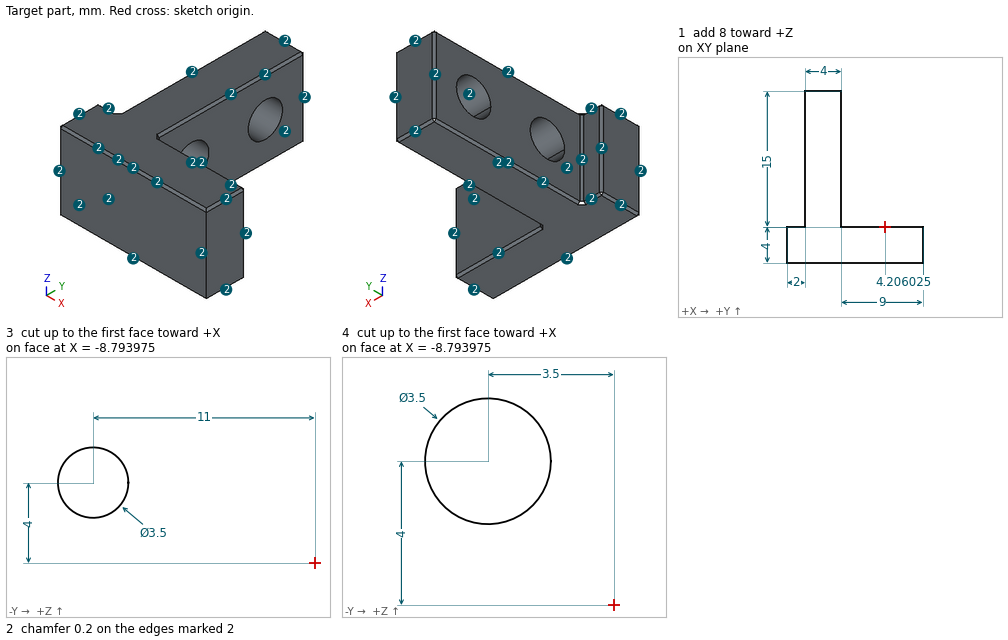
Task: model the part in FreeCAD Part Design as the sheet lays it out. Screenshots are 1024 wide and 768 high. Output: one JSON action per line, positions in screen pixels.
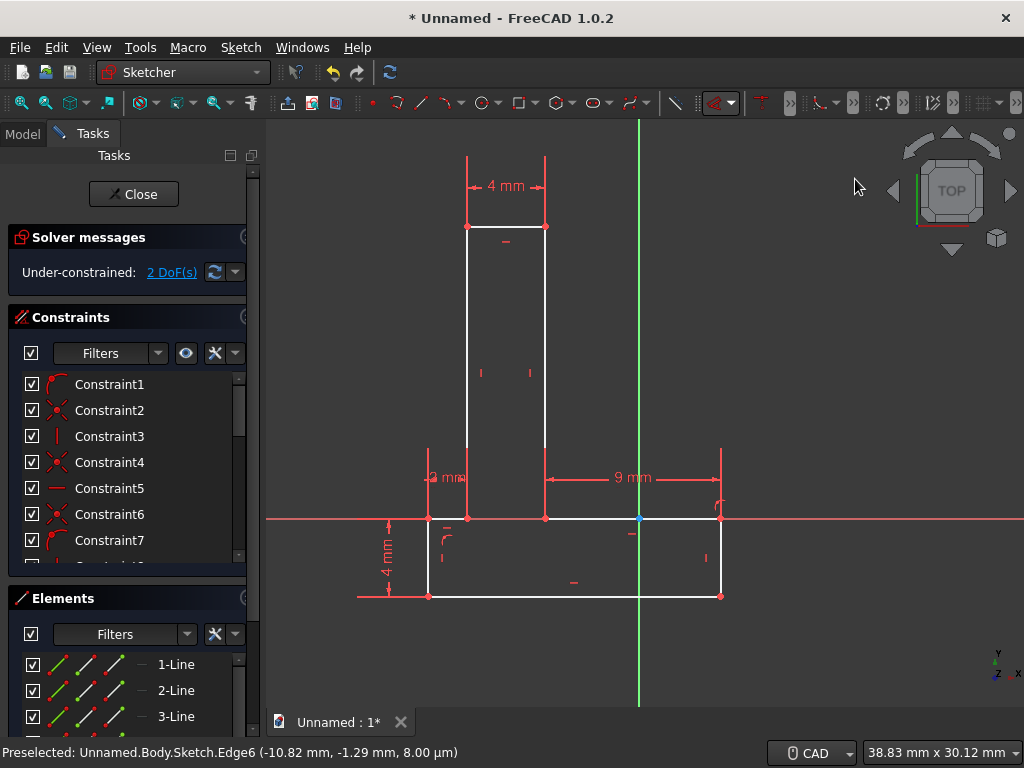
{"action": "left_click", "coordinate": [545, 431]}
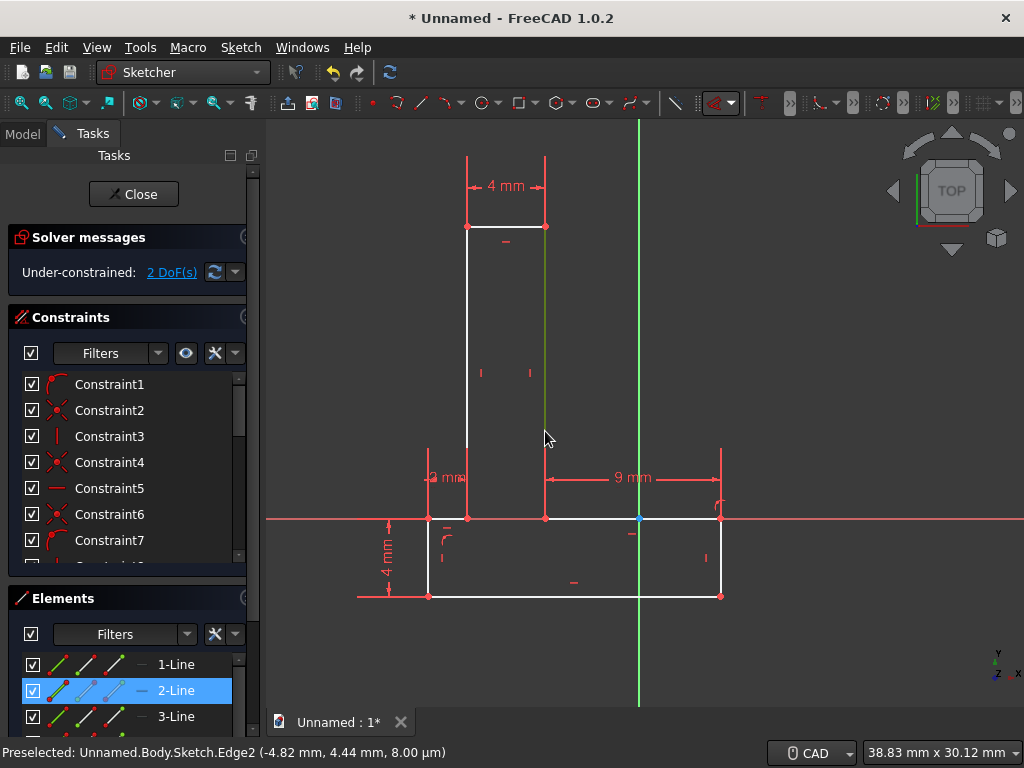
{"action": "left_click", "coordinate": [734, 104]}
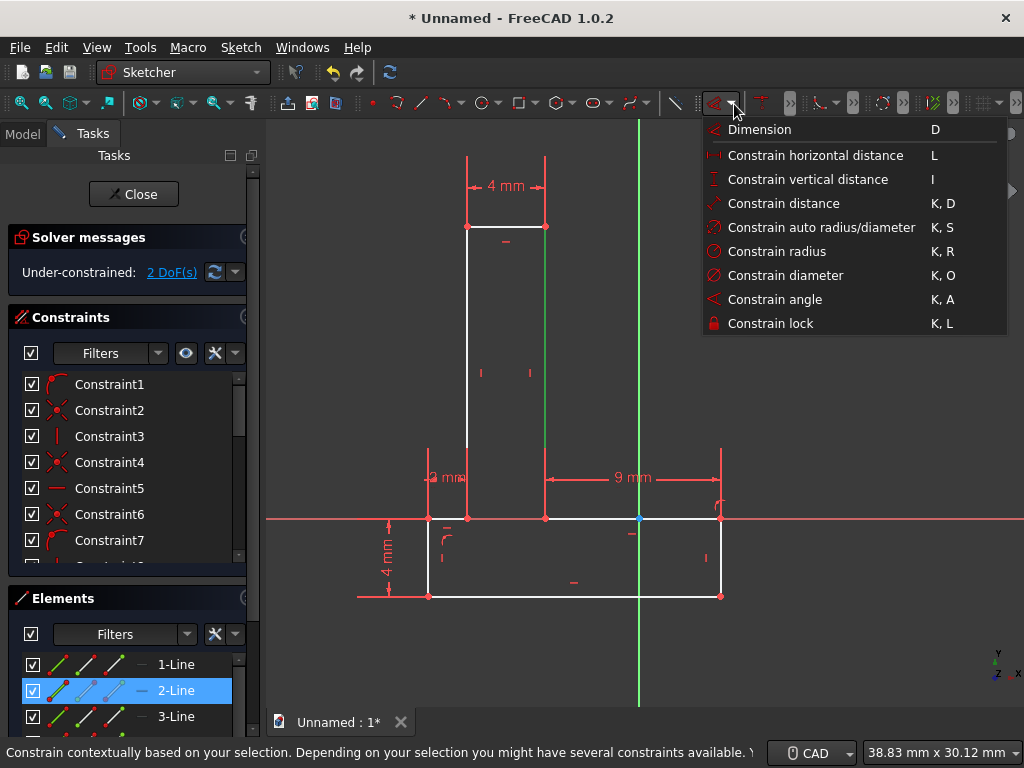
{"action": "left_click", "coordinate": [855, 179]}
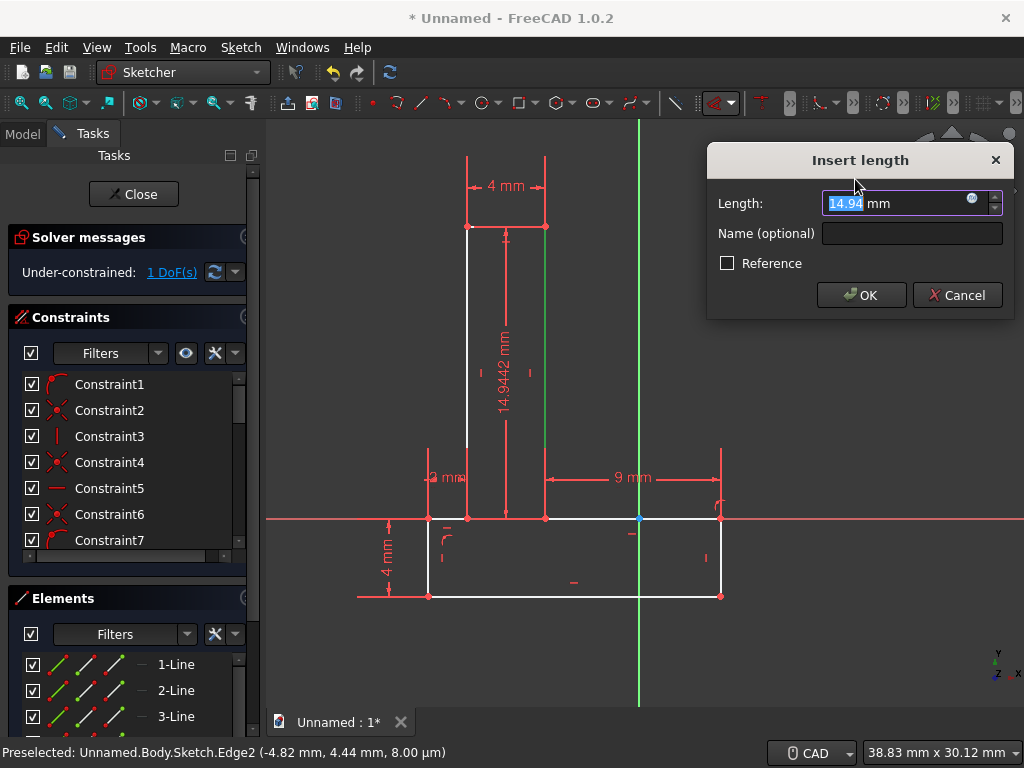
{"action": "type", "text": "15"}
{"action": "key", "text": "Return"}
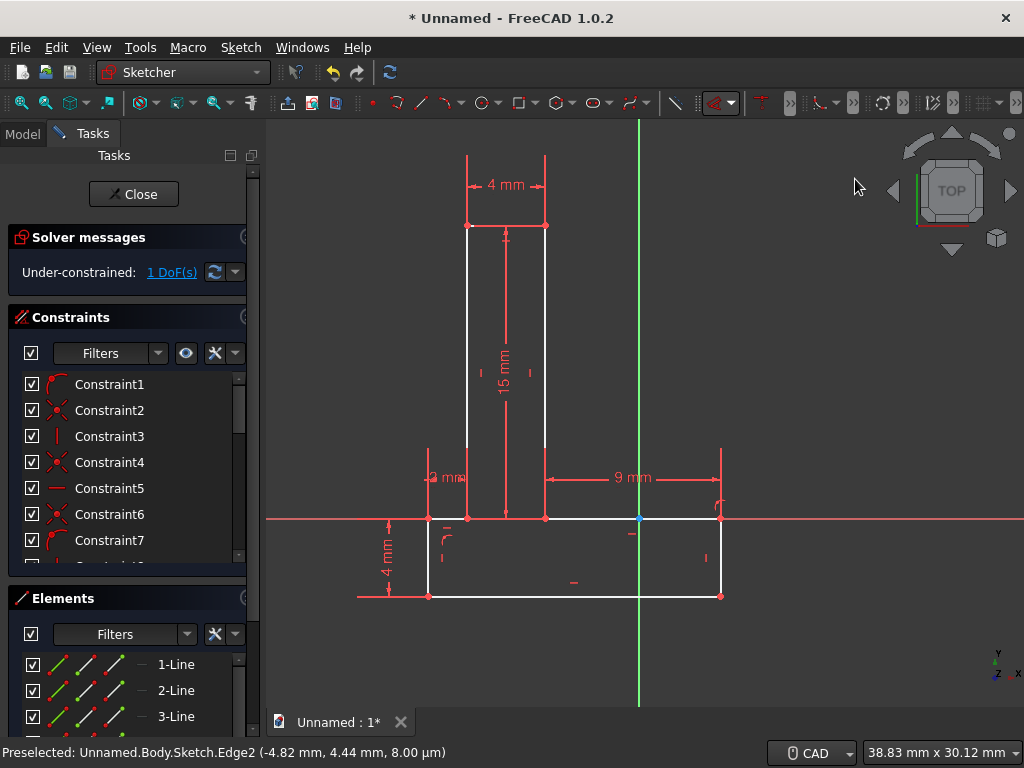
{"action": "left_click", "coordinate": [721, 519]}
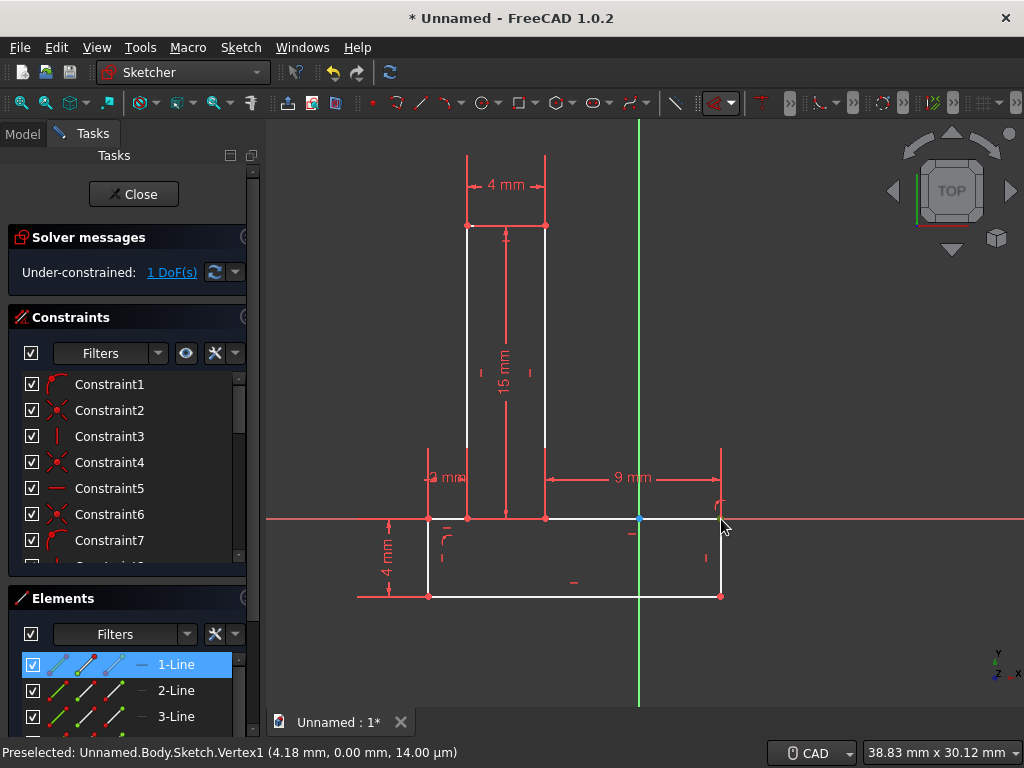
{"action": "key", "text": "l"}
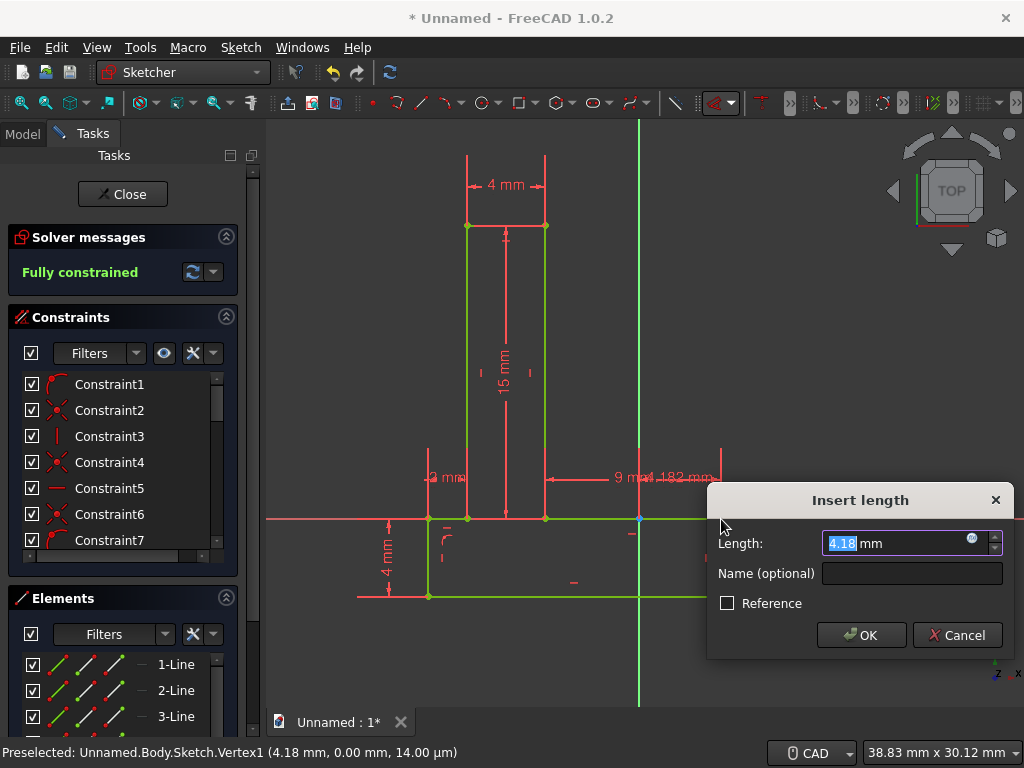
{"action": "type", "text": "4.206025"}
{"action": "key", "text": "Return"}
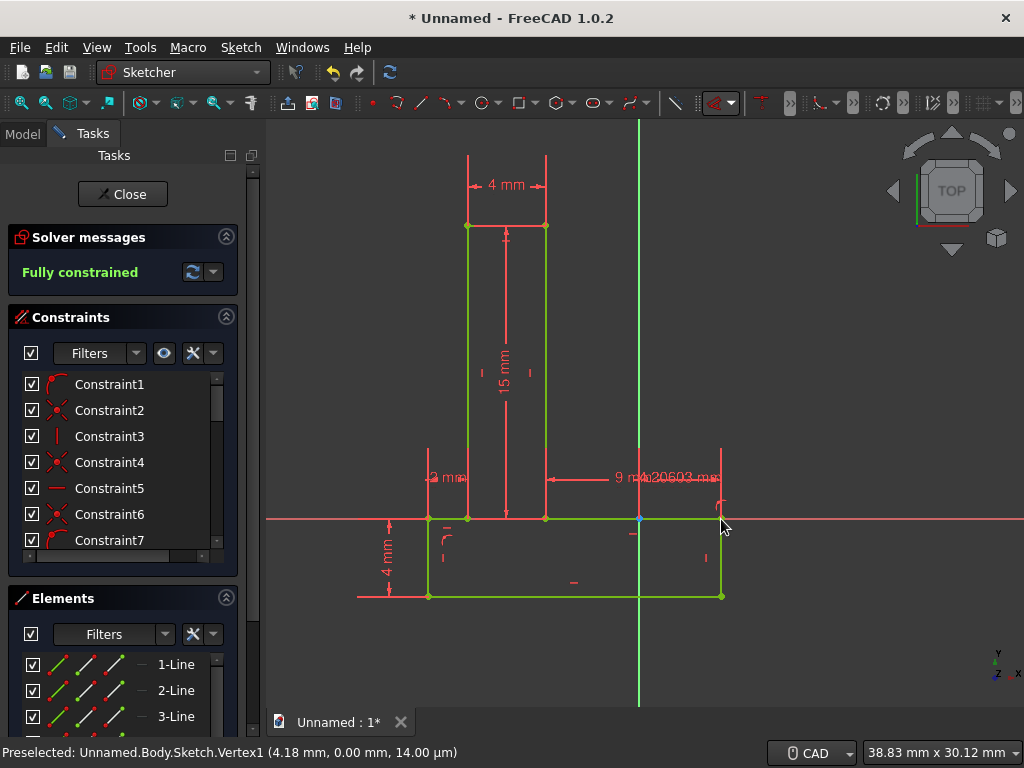
{"action": "left_click", "coordinate": [123, 194]}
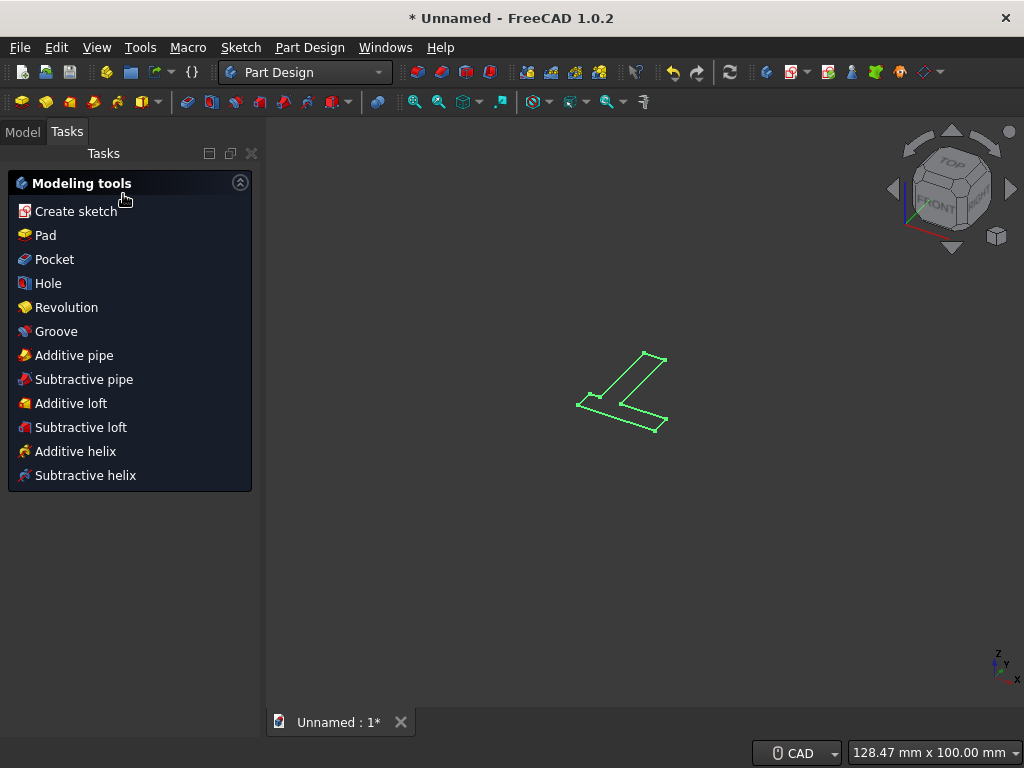
{"action": "left_click", "coordinate": [22, 102]}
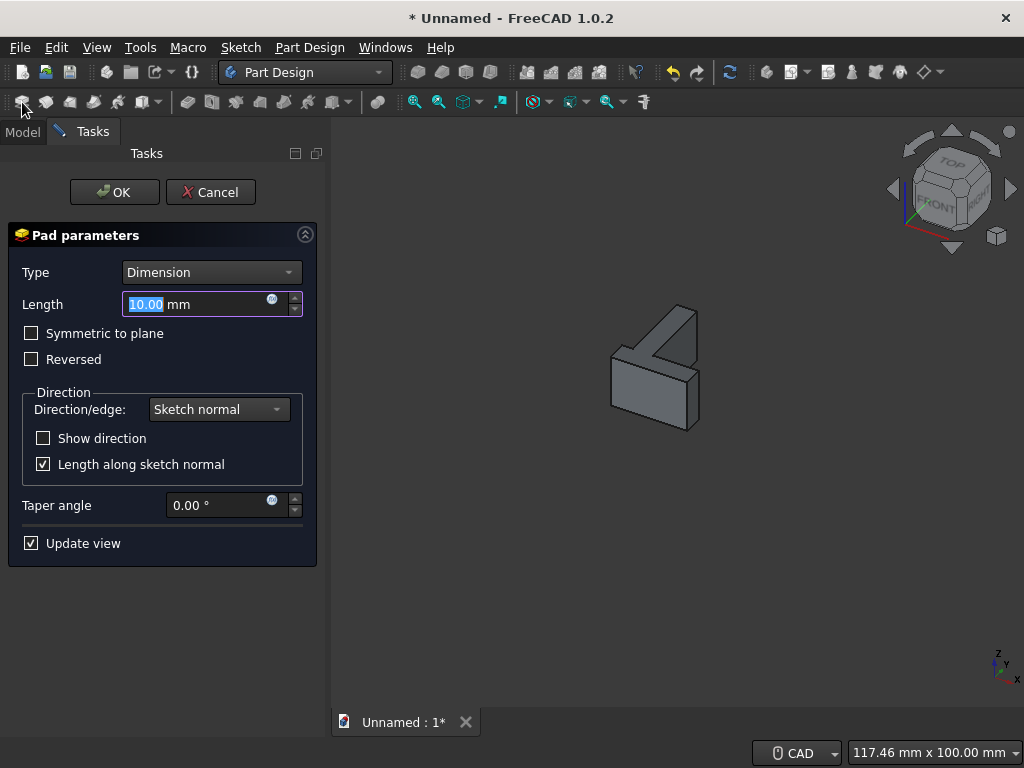
{"action": "type", "text": "8"}
{"action": "key", "text": "Tab"}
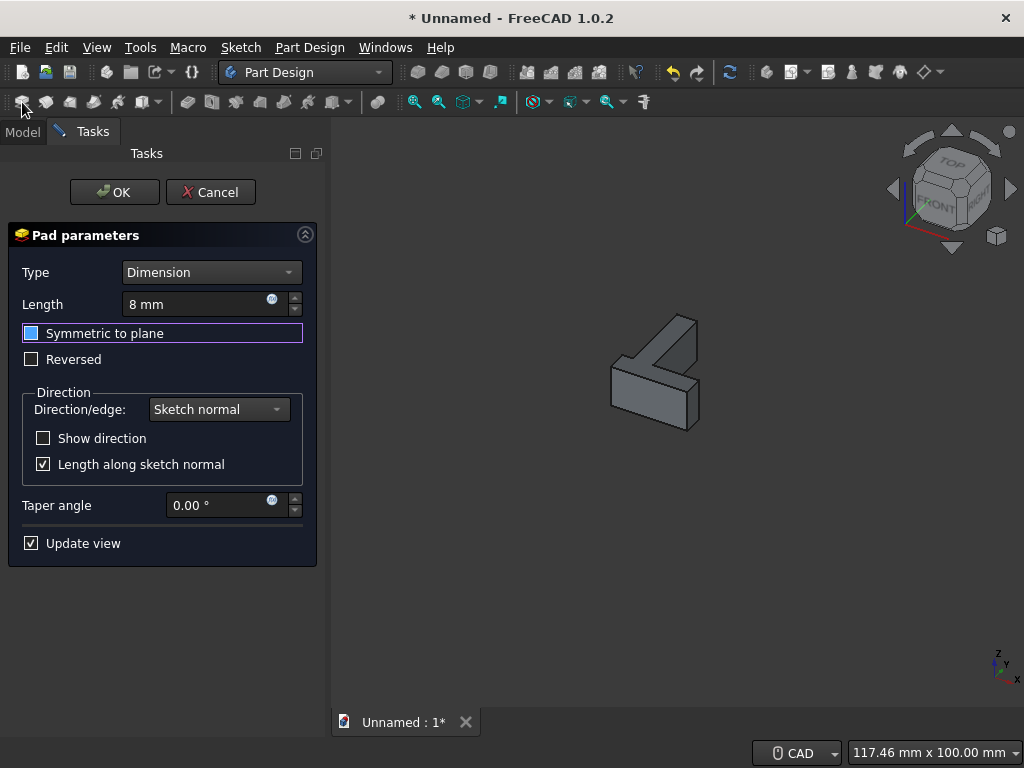
{"action": "left_click", "coordinate": [115, 192]}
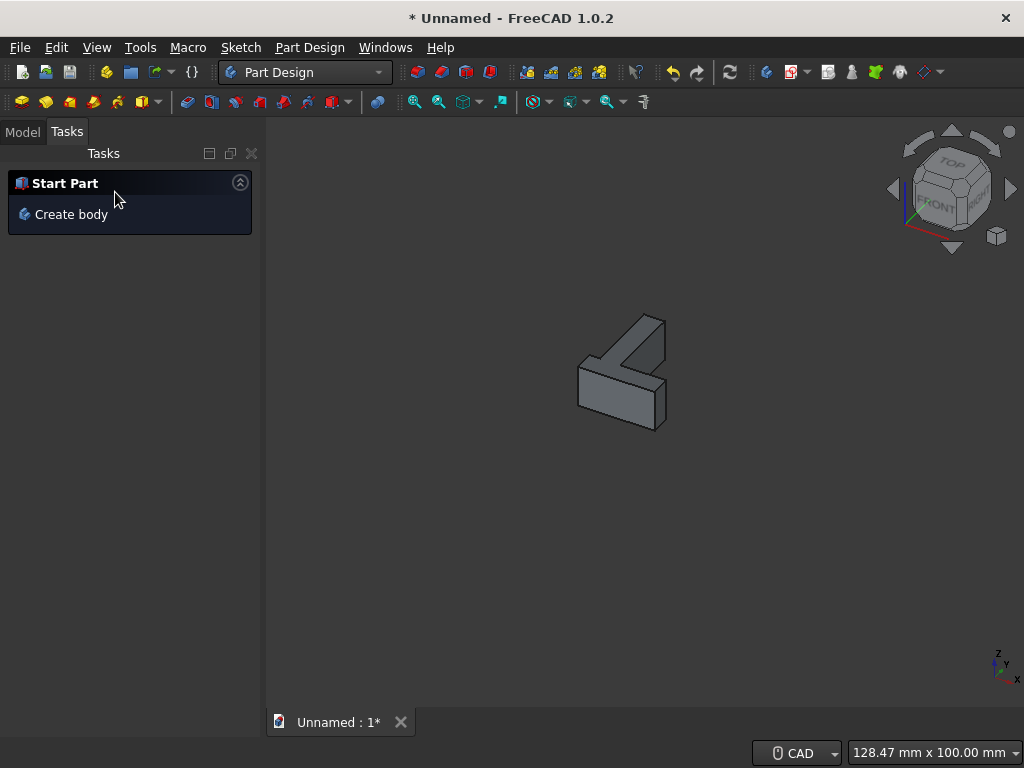
{"action": "left_click", "coordinate": [416, 102]}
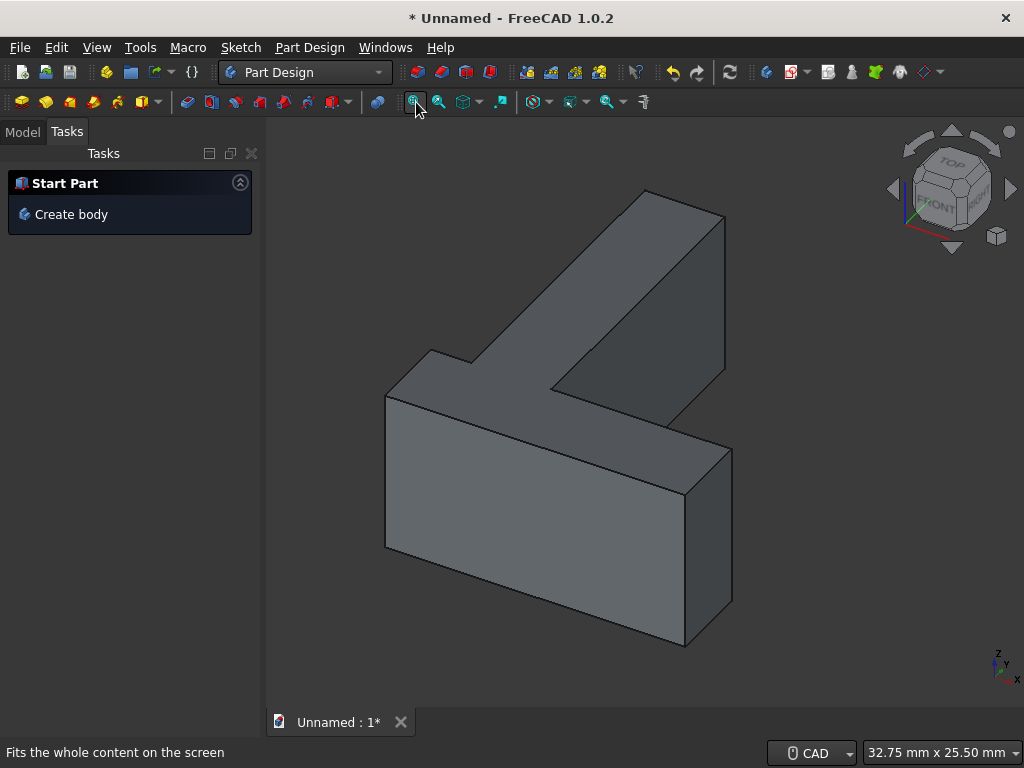
{"action": "left_click", "coordinate": [663, 353]}